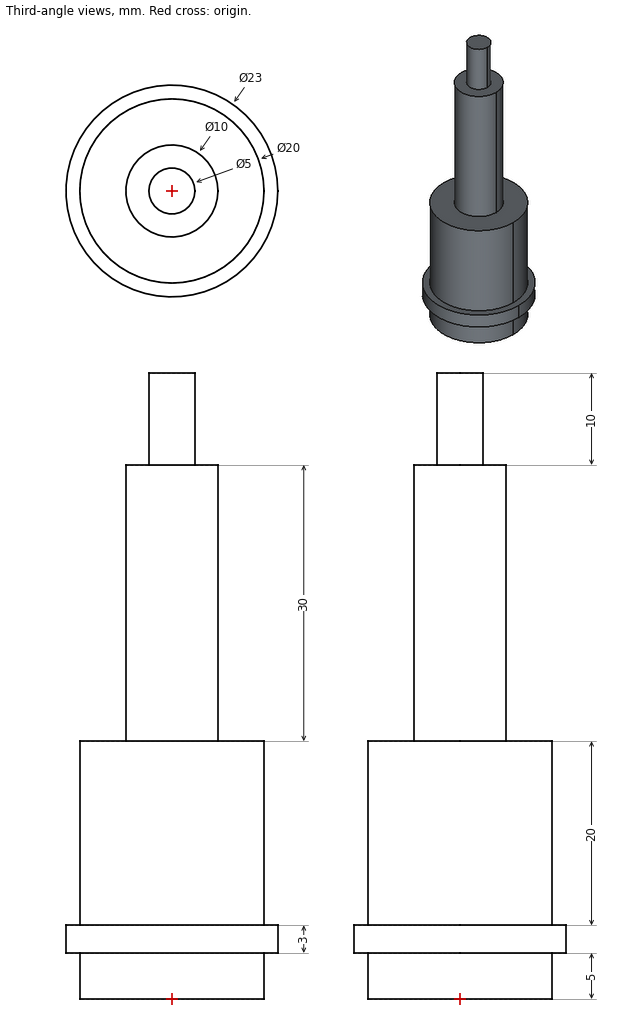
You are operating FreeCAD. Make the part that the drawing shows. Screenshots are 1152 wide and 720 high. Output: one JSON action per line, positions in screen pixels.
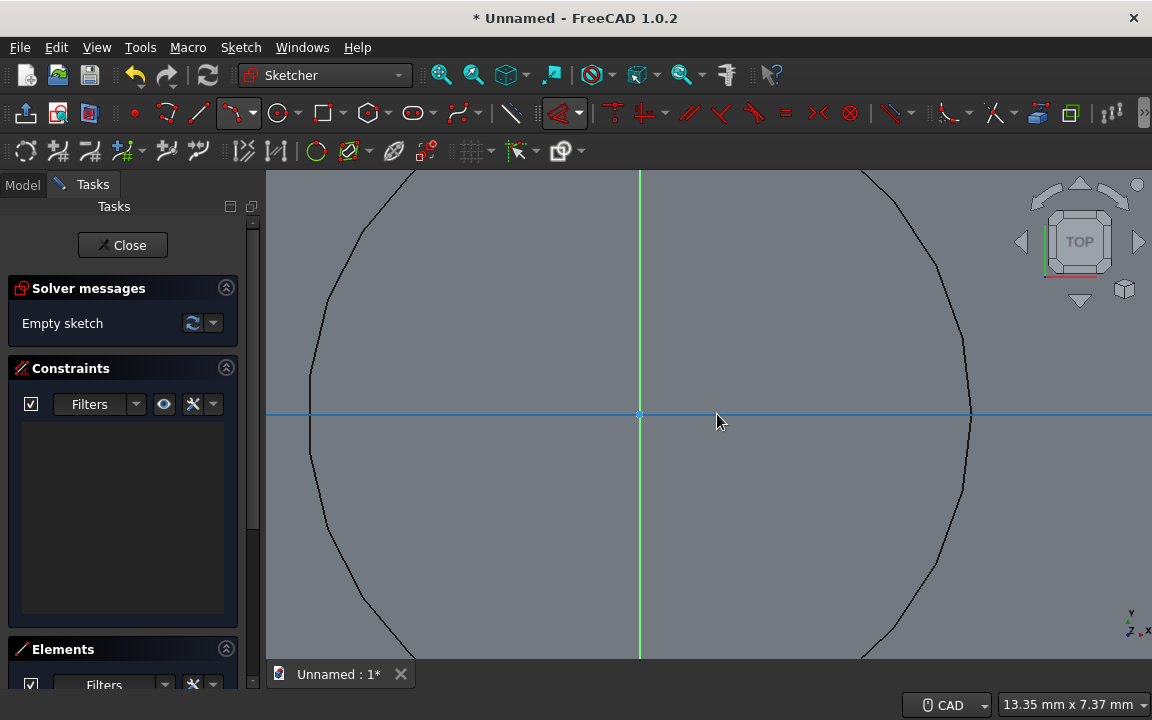
{"action": "left_click", "coordinate": [278, 114]}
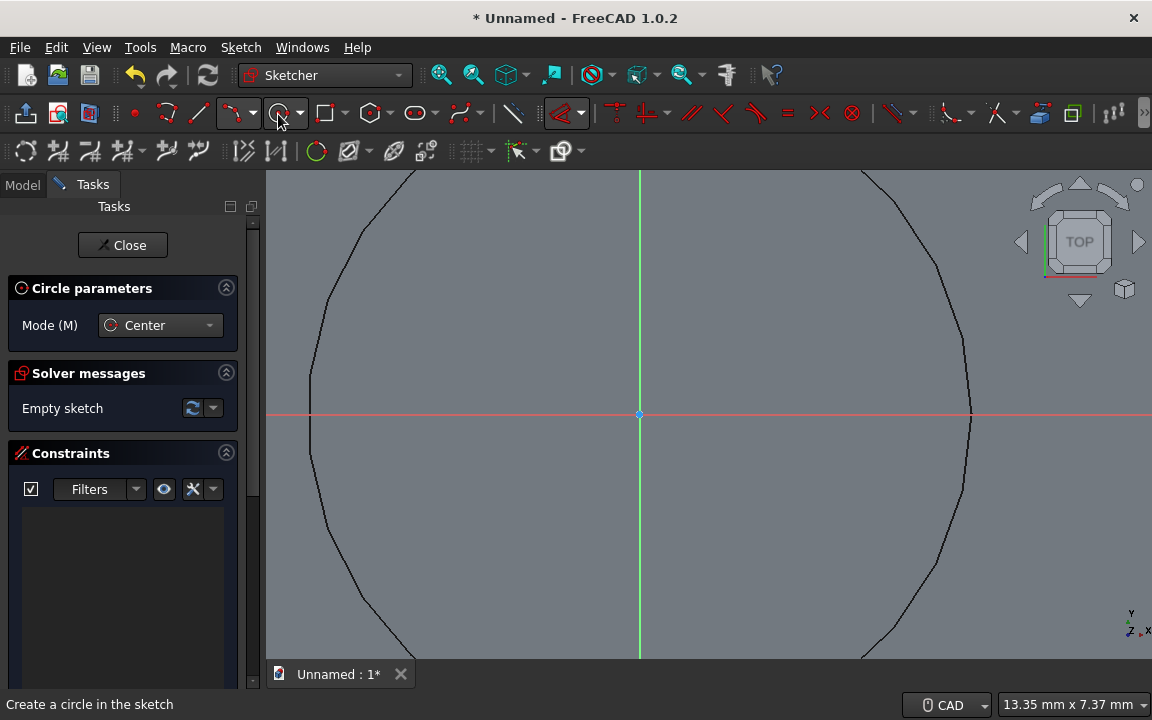
{"action": "left_click", "coordinate": [640, 414]}
{"action": "mouse_move", "coordinate": [757, 297]}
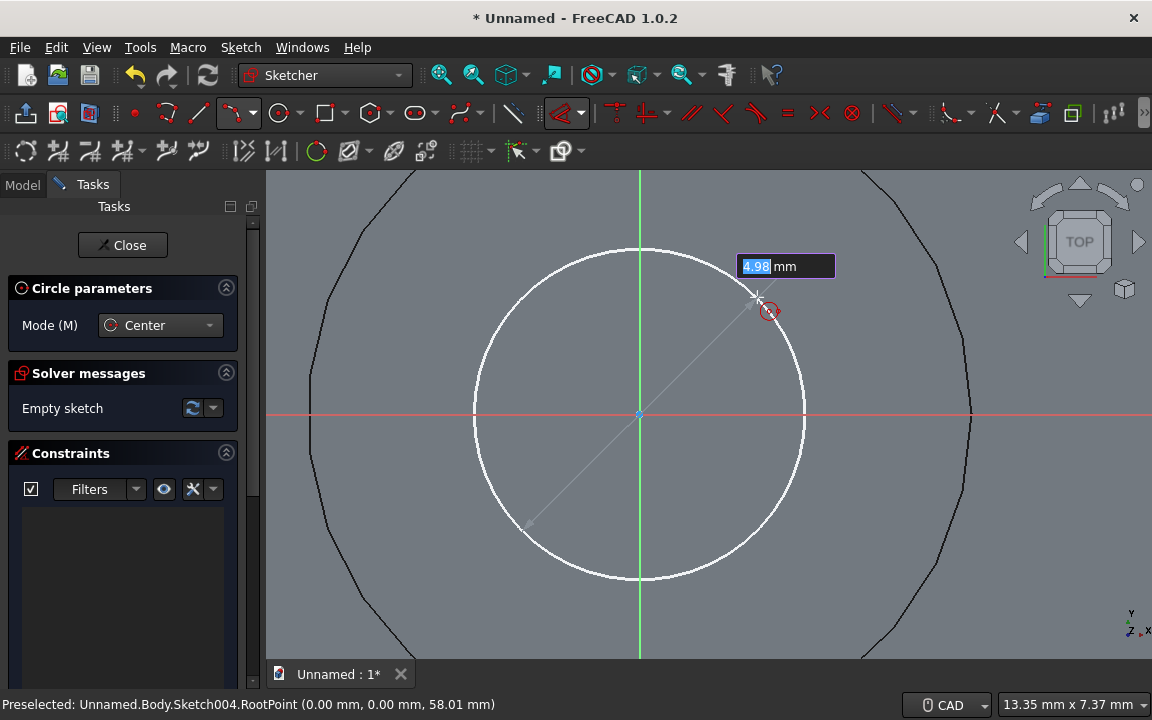
{"action": "type", "text": "5"}
{"action": "key", "text": "Return"}
{"action": "key", "text": "Escape"}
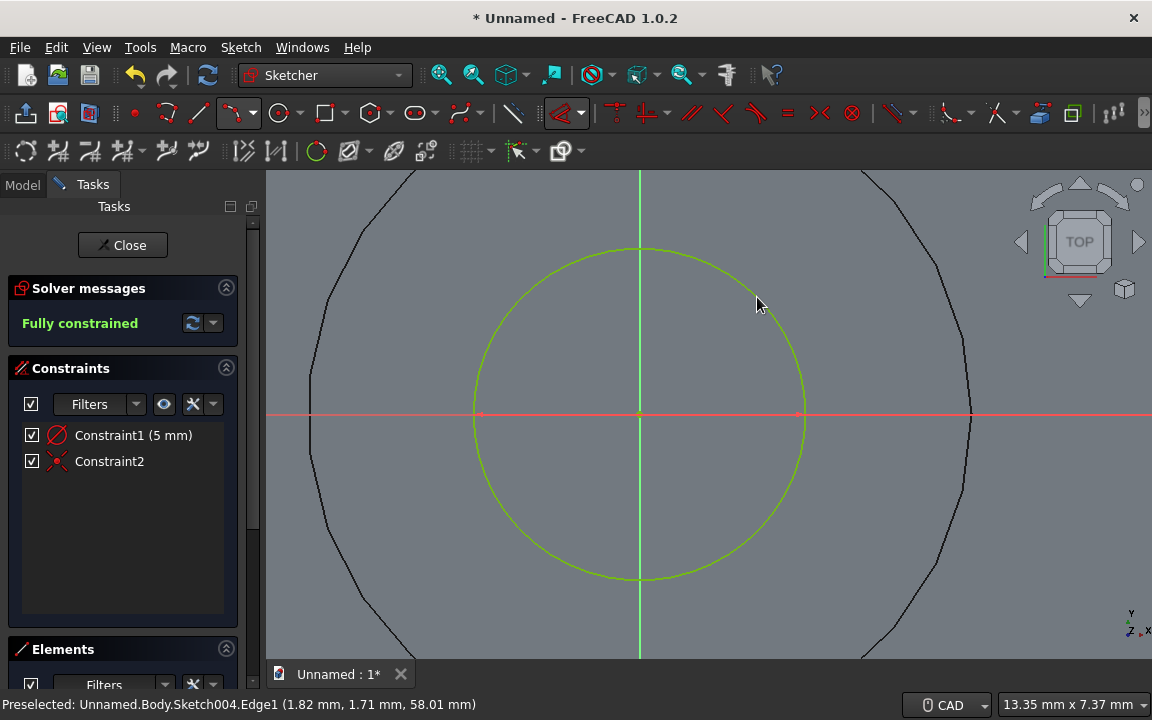
{"action": "left_click", "coordinate": [123, 245]}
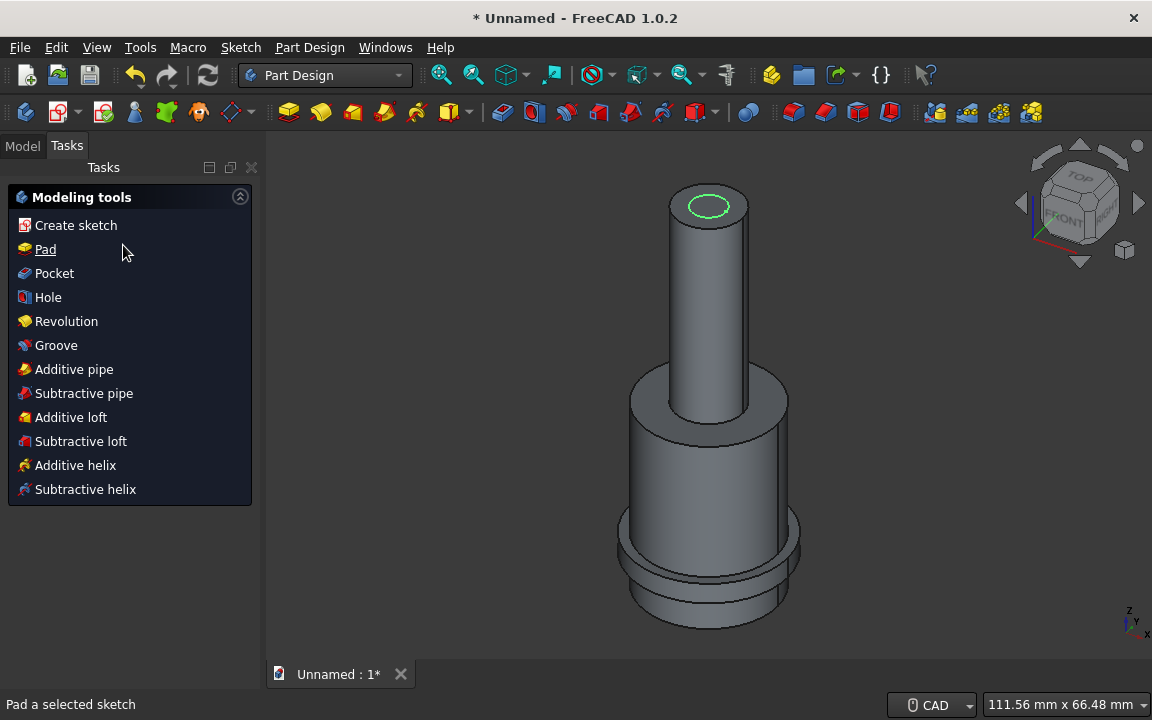
{"action": "left_click", "coordinate": [290, 112]}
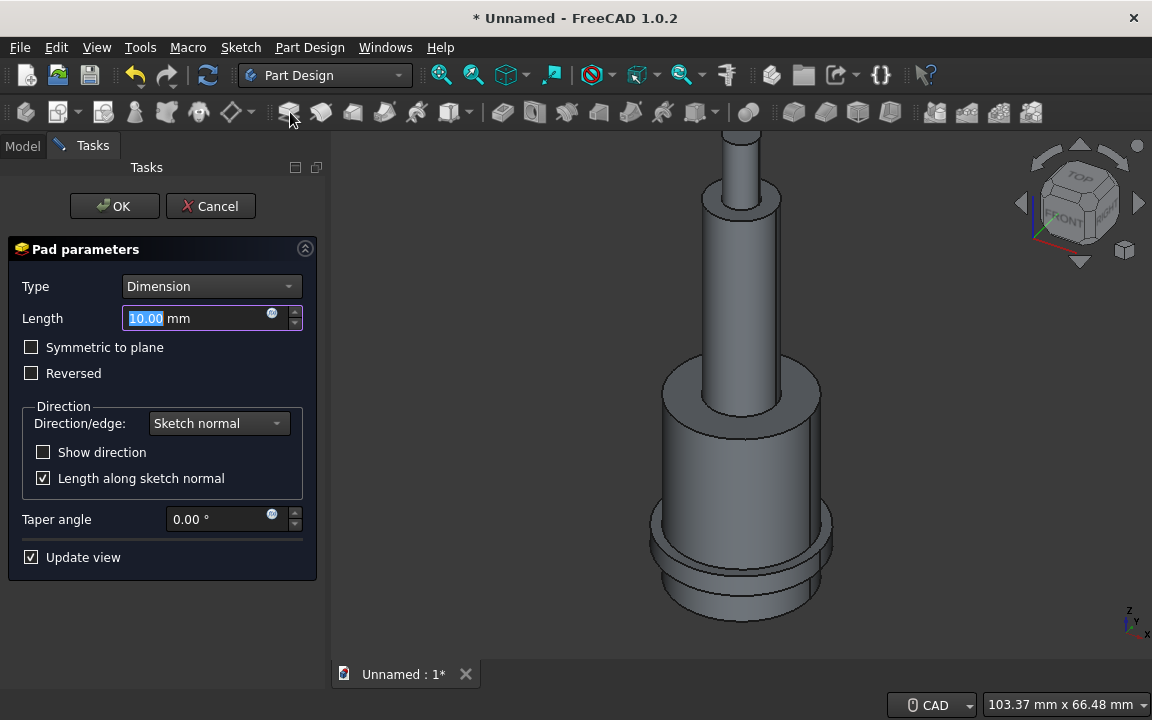
{"action": "type", "text": "10"}
{"action": "key", "text": "Tab"}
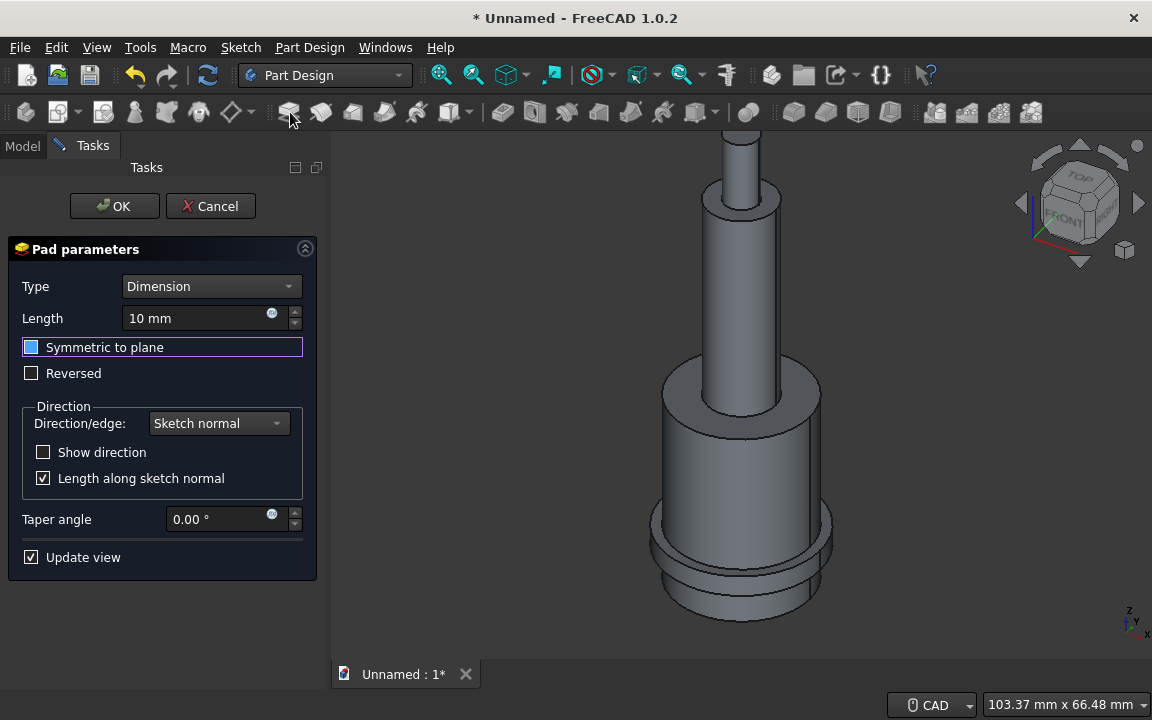
{"action": "left_click", "coordinate": [115, 206]}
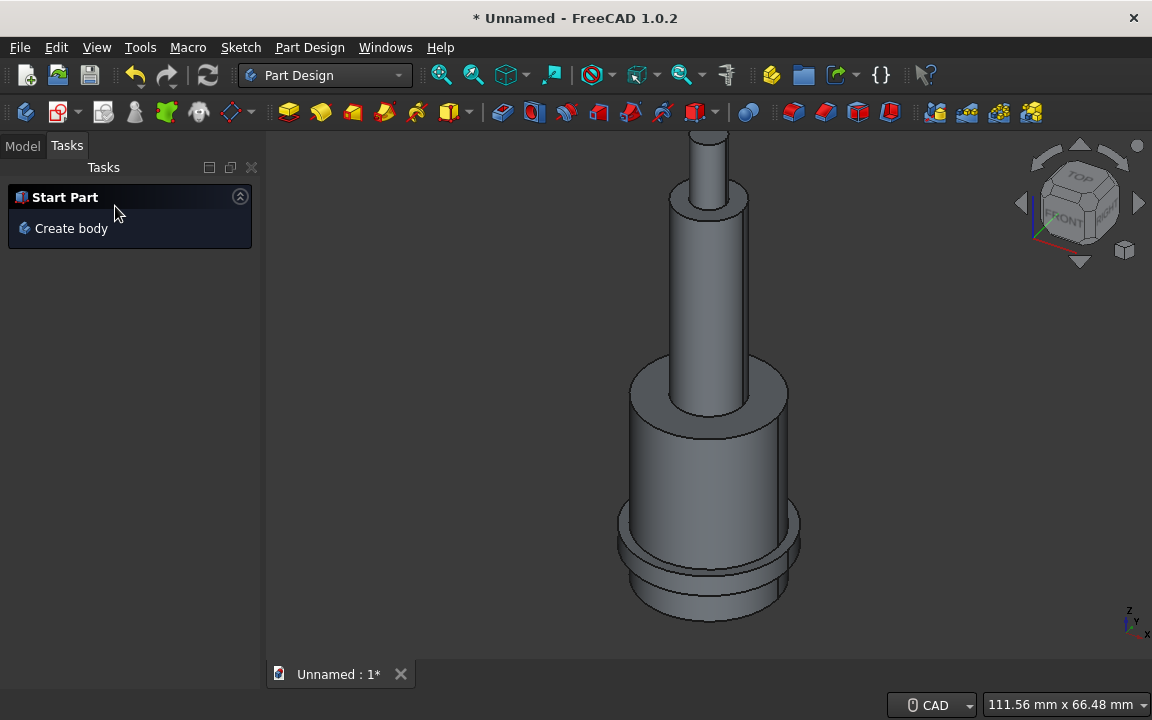
{"action": "key", "text": "0"}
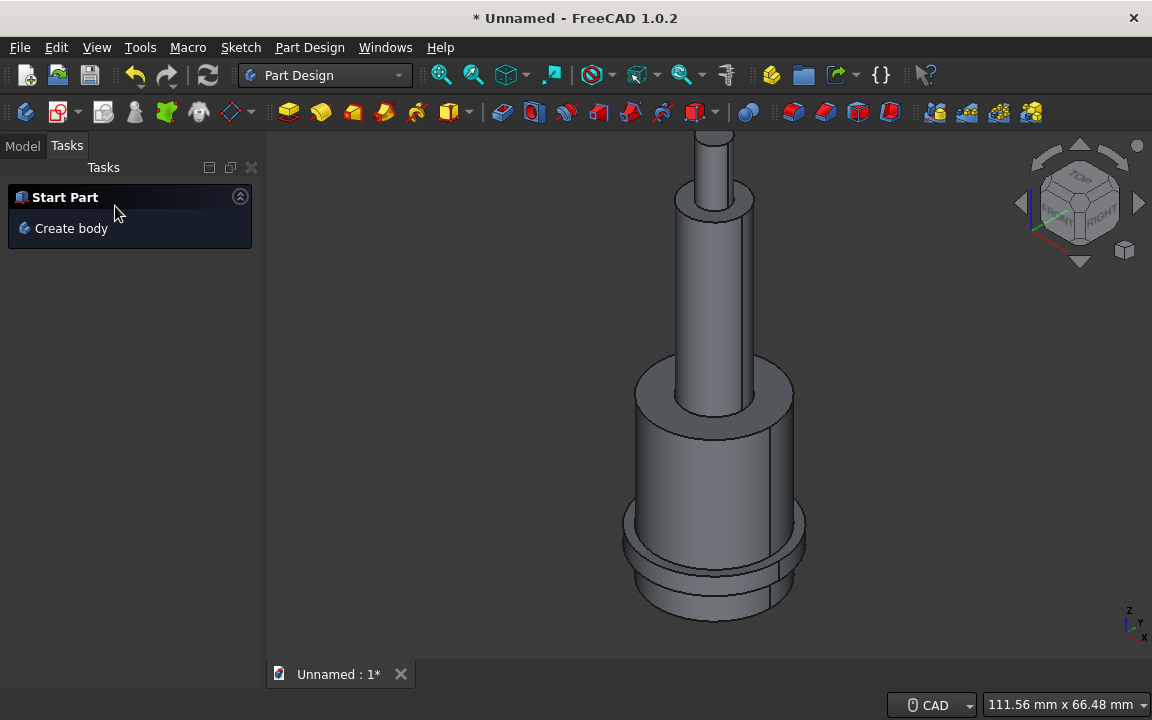
{"action": "left_click", "coordinate": [442, 76]}